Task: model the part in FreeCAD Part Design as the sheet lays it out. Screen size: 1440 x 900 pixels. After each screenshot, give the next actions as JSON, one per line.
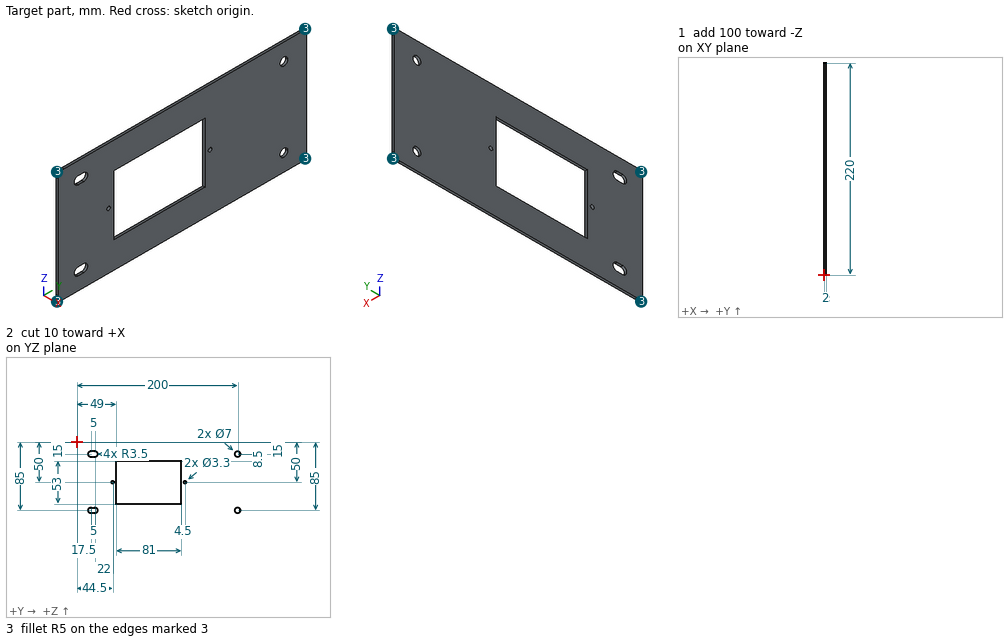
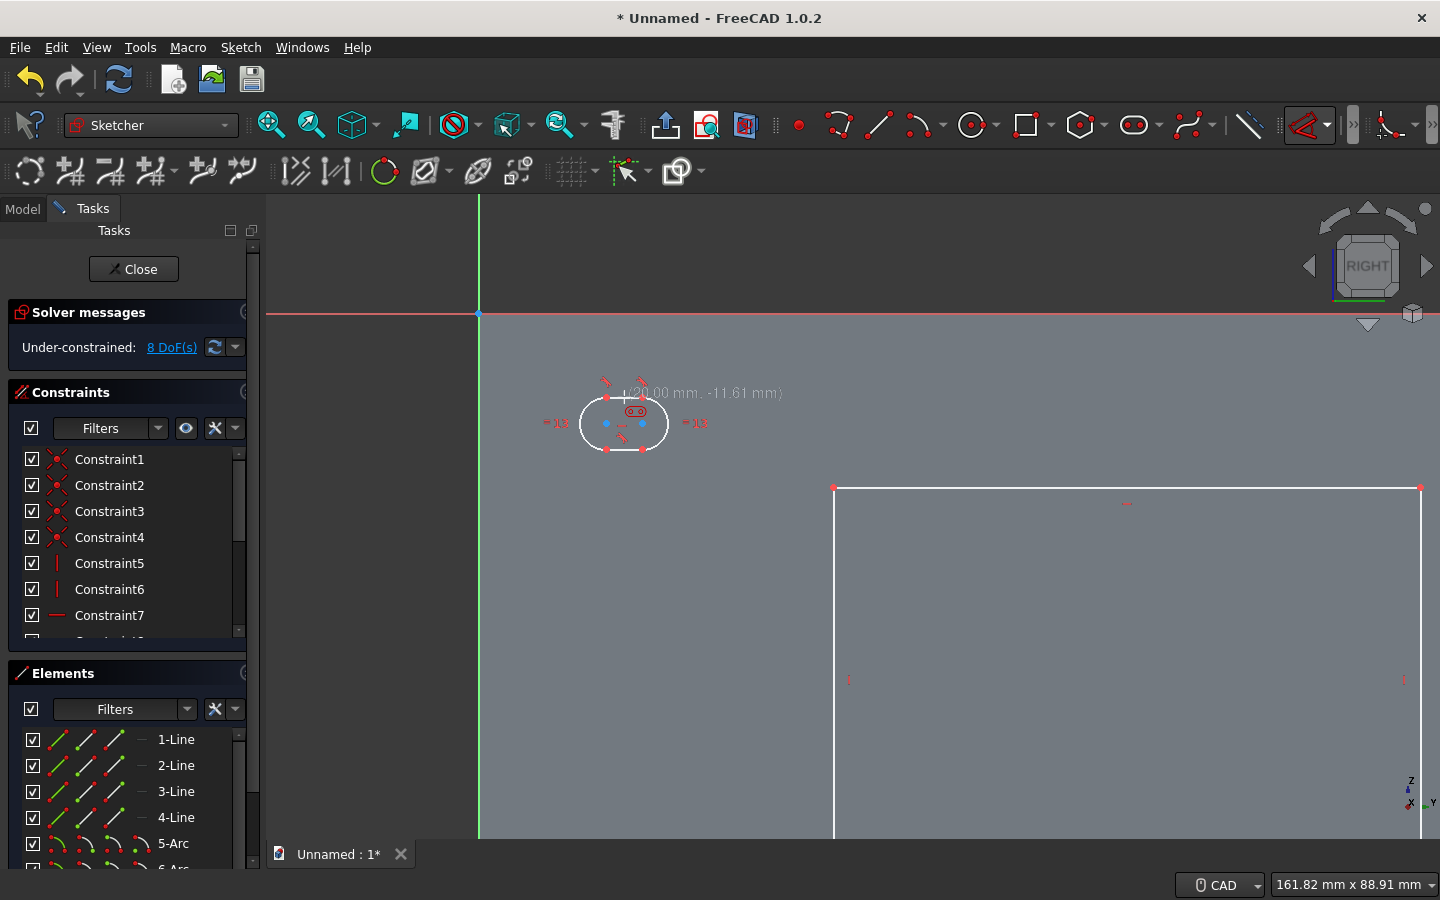
{"action": "scroll", "coordinate": [432, 420], "scroll_direction": "down", "scroll_amount": 4}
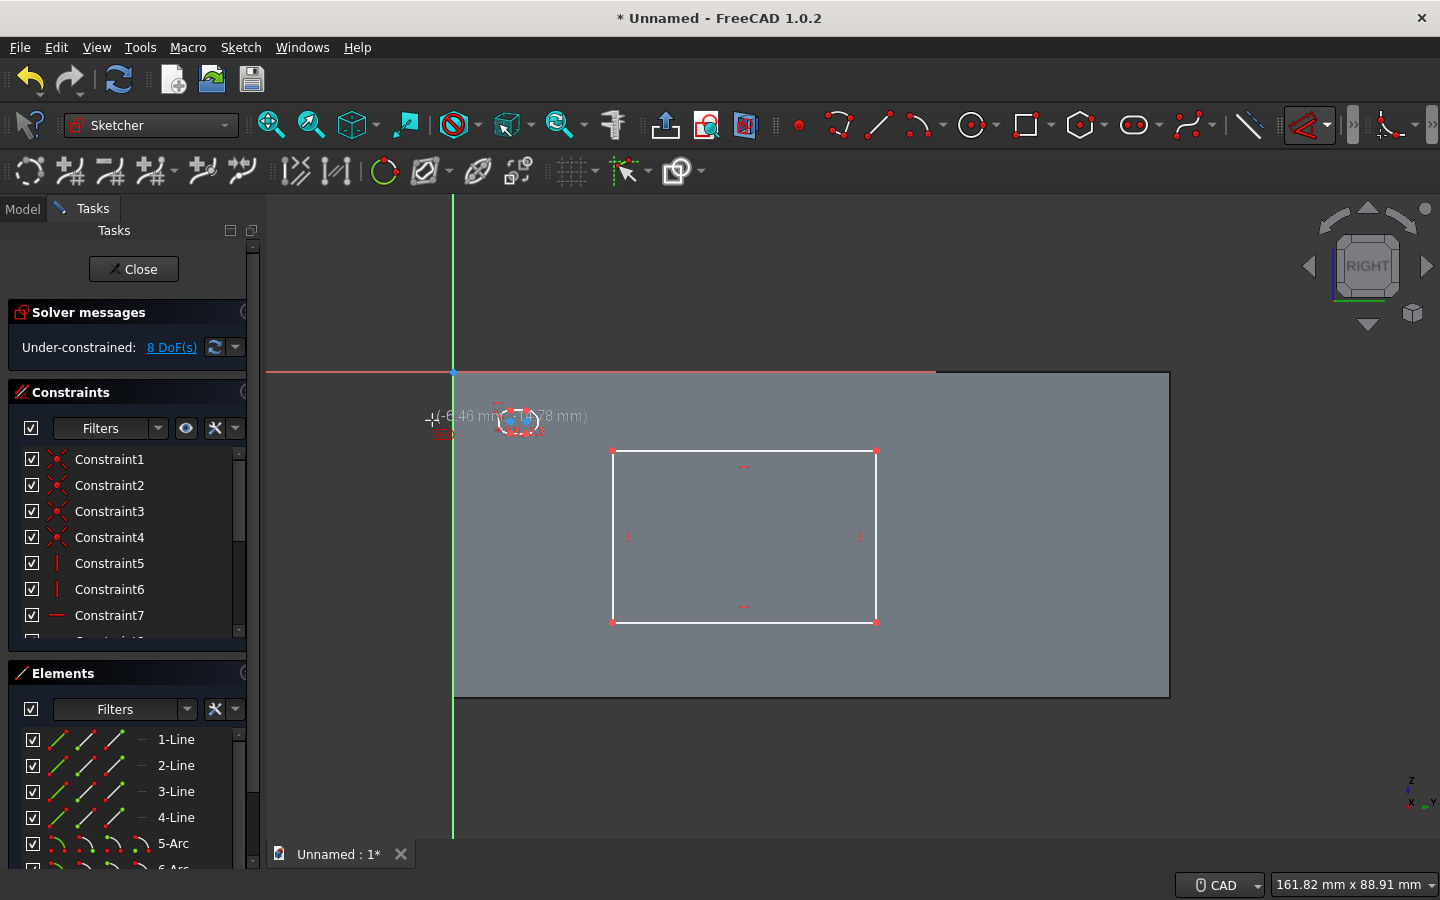
{"action": "scroll", "coordinate": [510, 650], "scroll_direction": "up", "scroll_amount": 4}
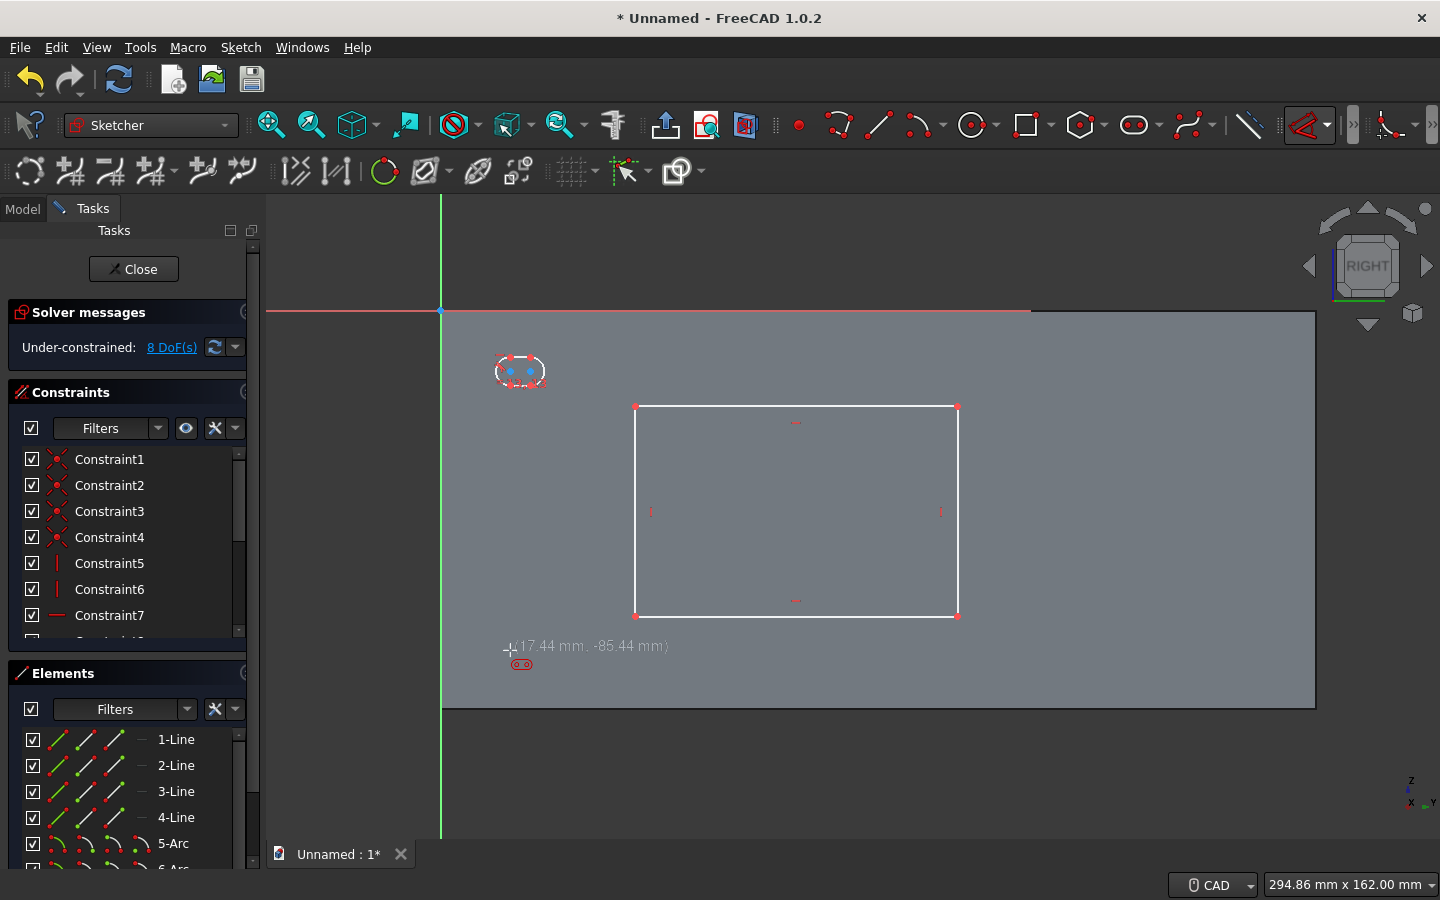
{"action": "left_click", "coordinate": [510, 648]}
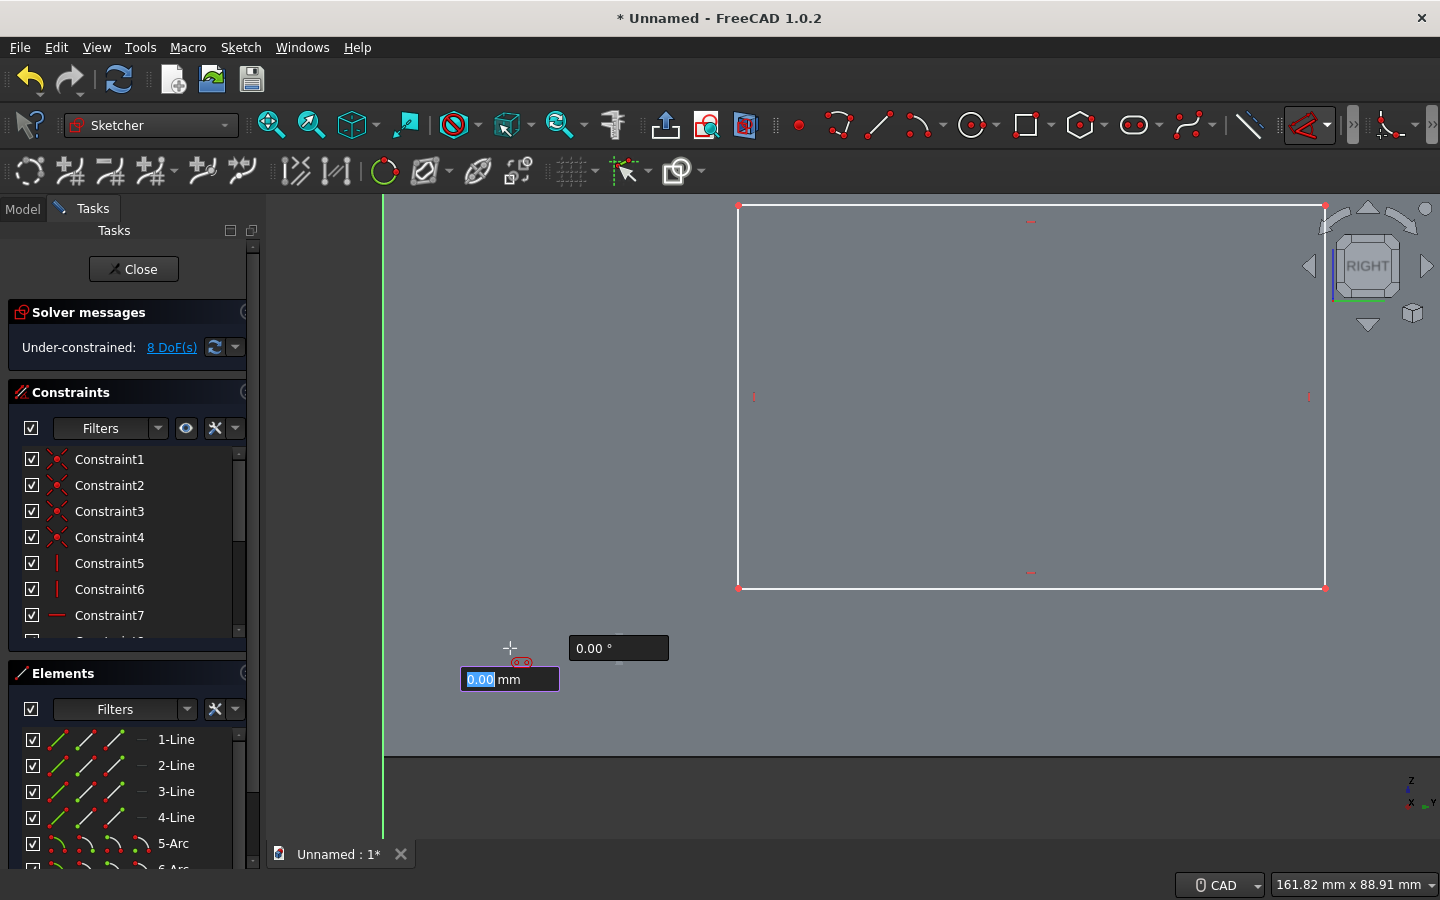
{"action": "left_click", "coordinate": [546, 648]}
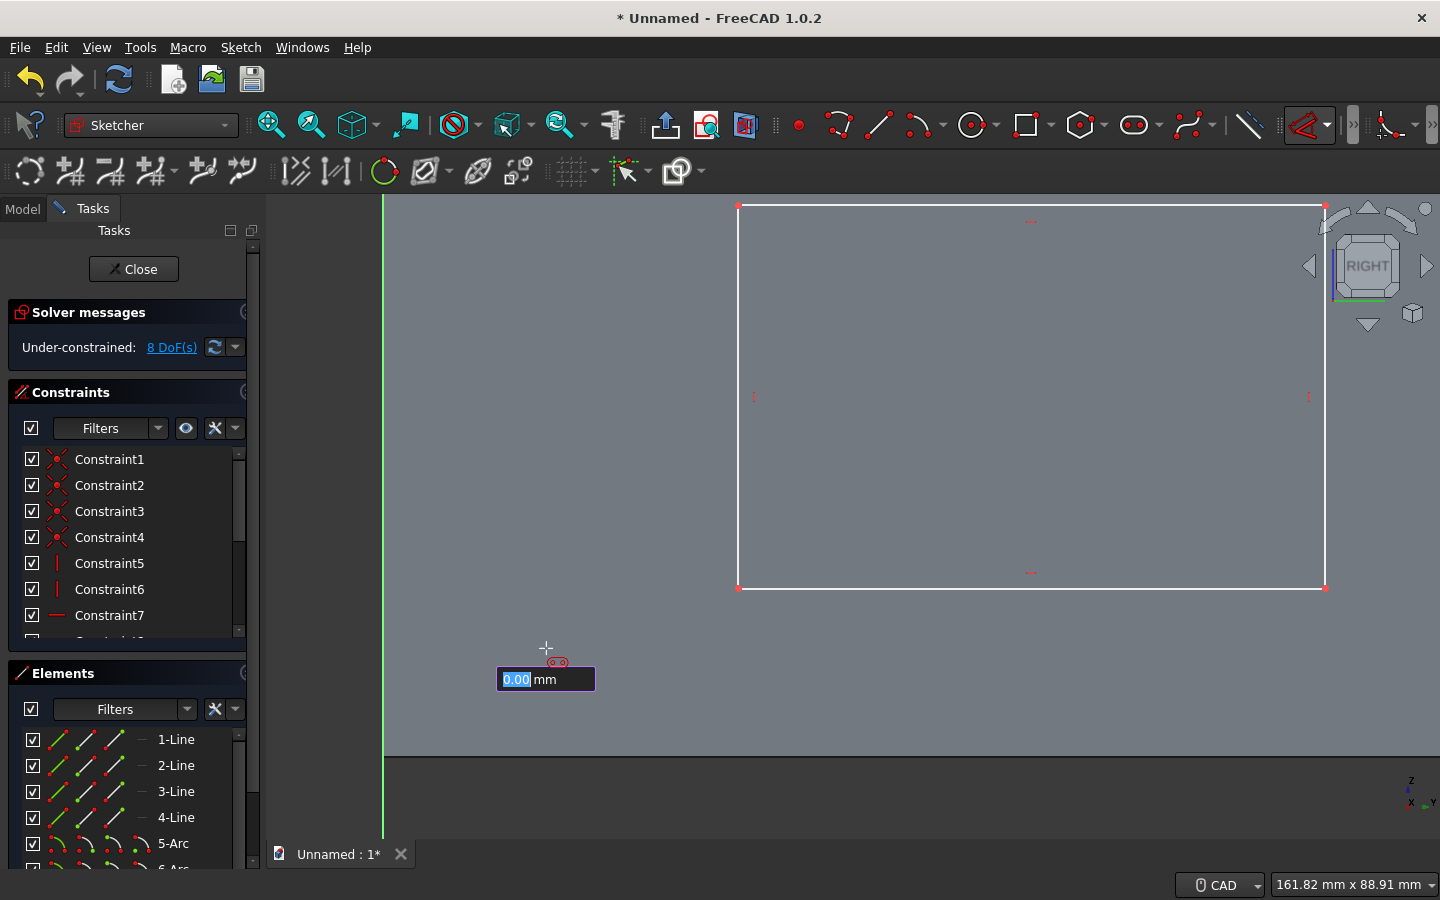
{"action": "left_click", "coordinate": [528, 623]}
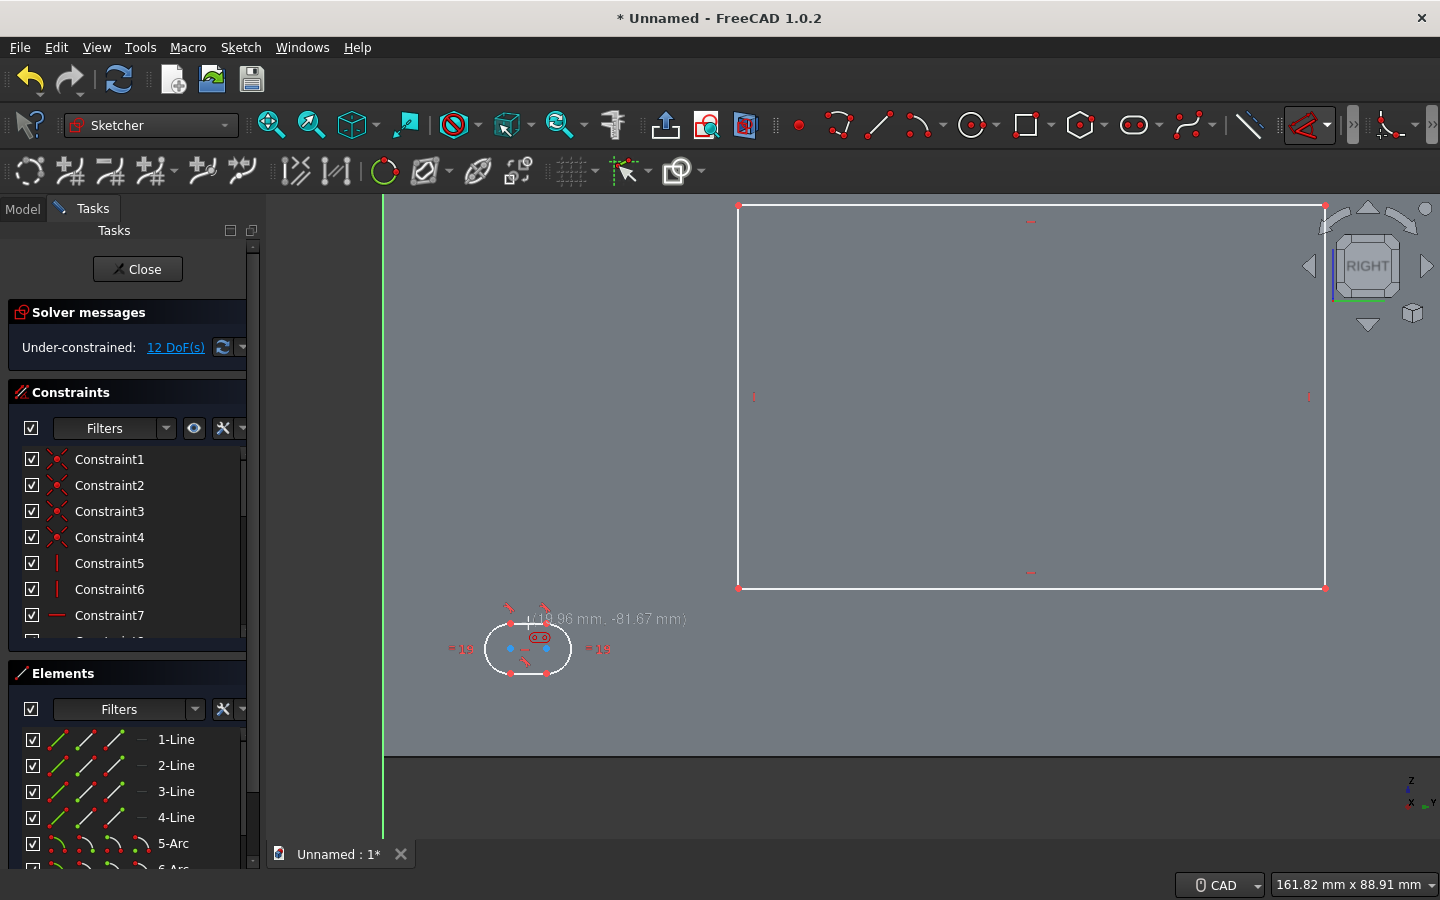
{"action": "left_click", "coordinate": [972, 126]}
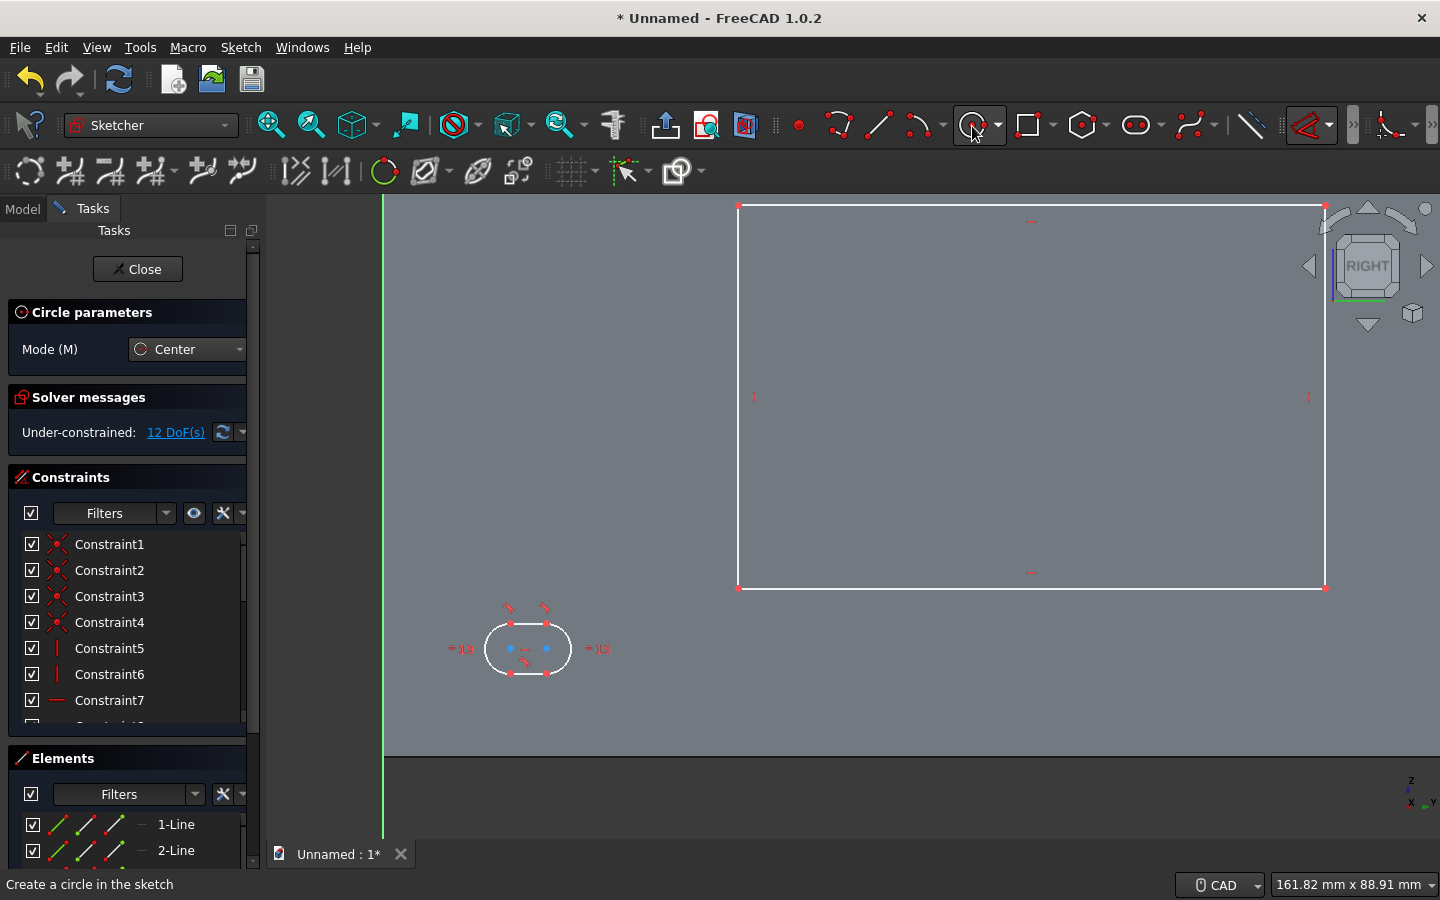
{"action": "scroll", "coordinate": [706, 394], "scroll_direction": "up", "scroll_amount": 4}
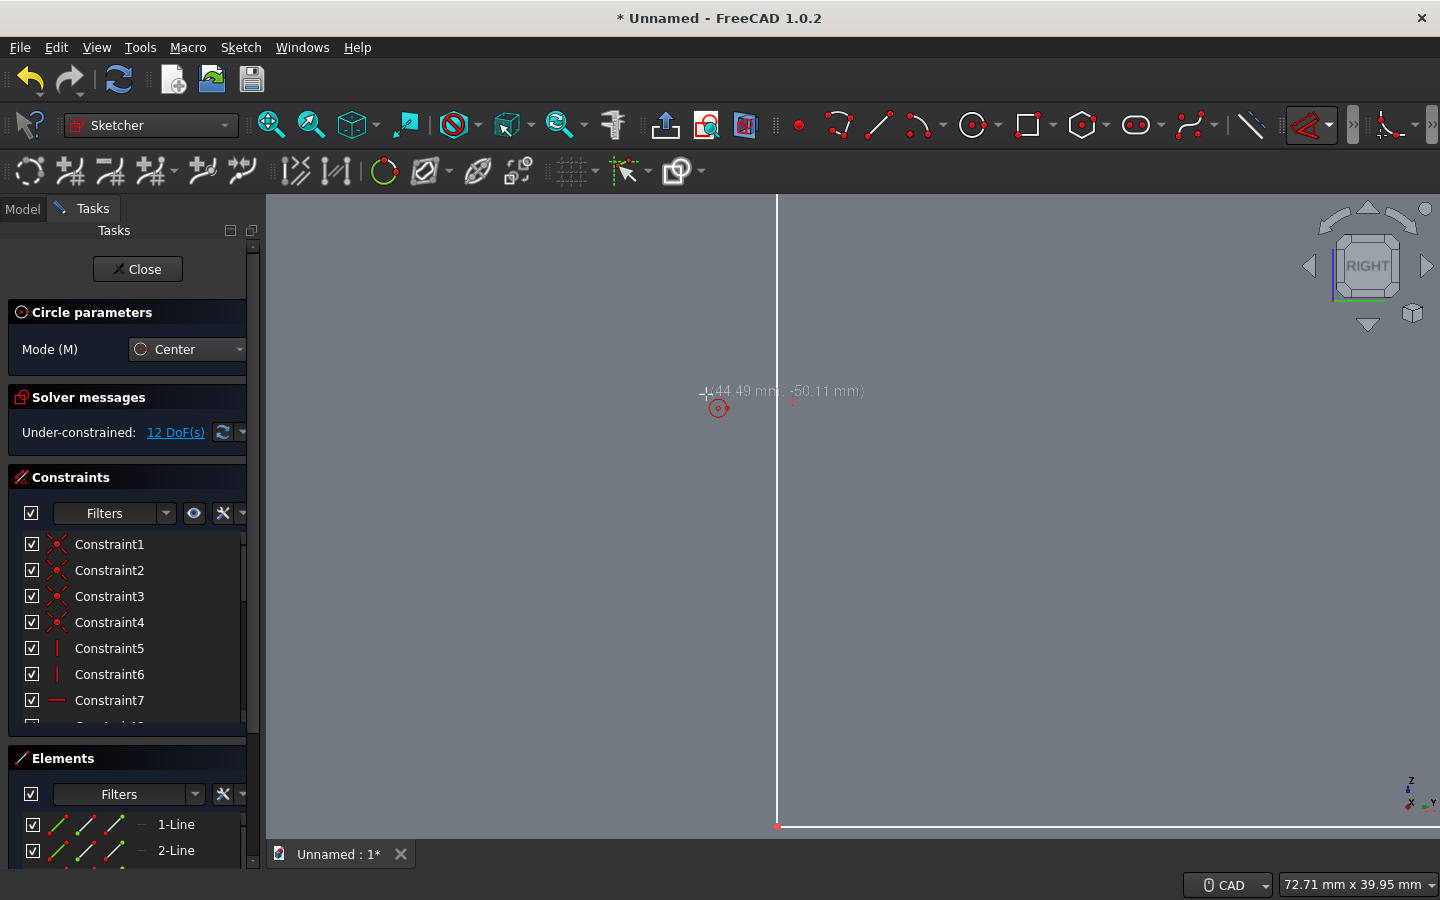
{"action": "scroll", "coordinate": [571, 571], "scroll_direction": "down", "scroll_amount": 8}